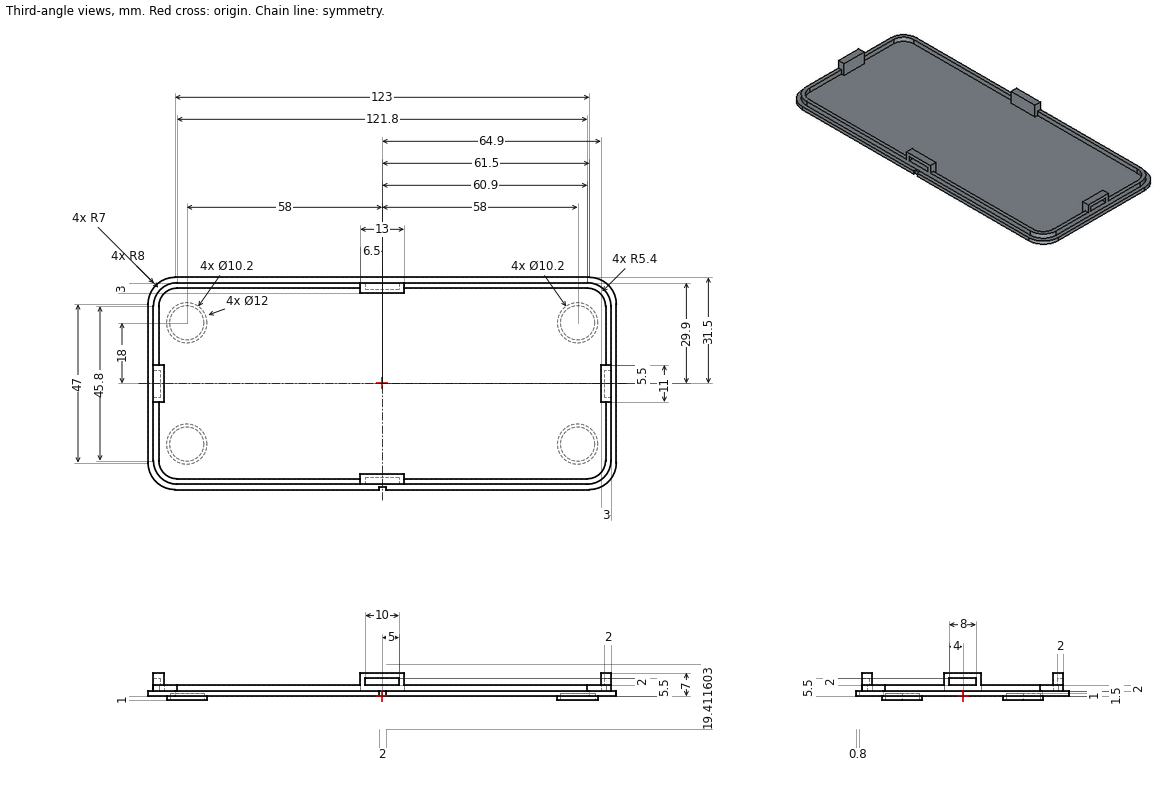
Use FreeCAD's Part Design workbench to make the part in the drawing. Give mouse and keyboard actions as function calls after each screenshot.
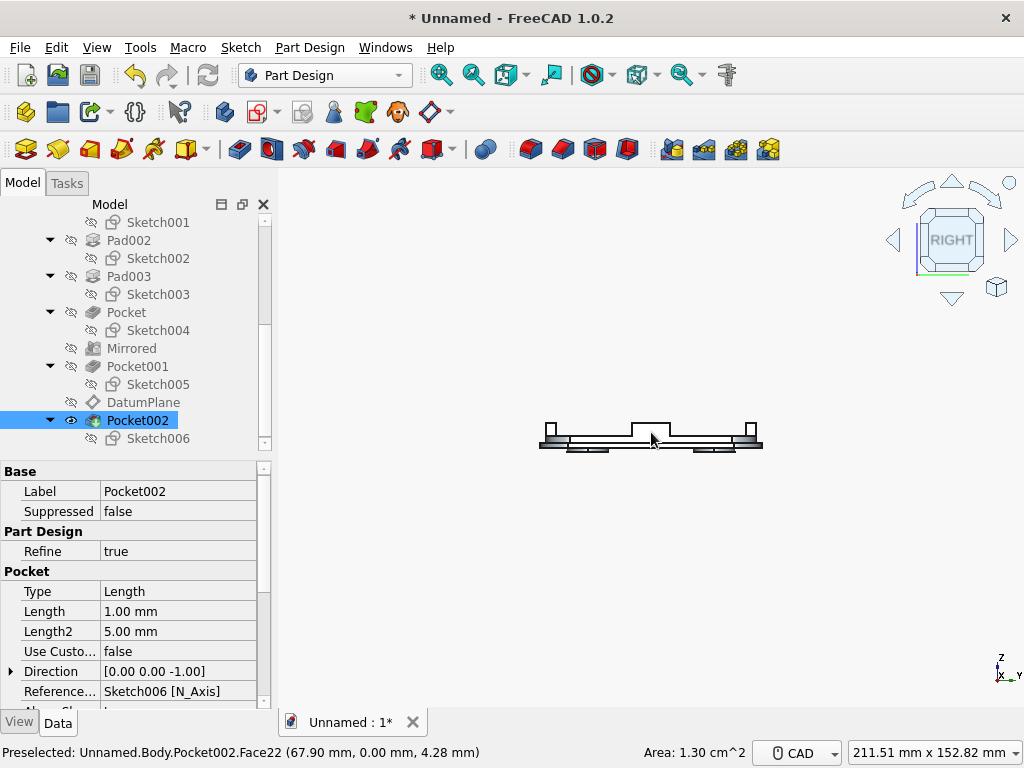
click(258, 112)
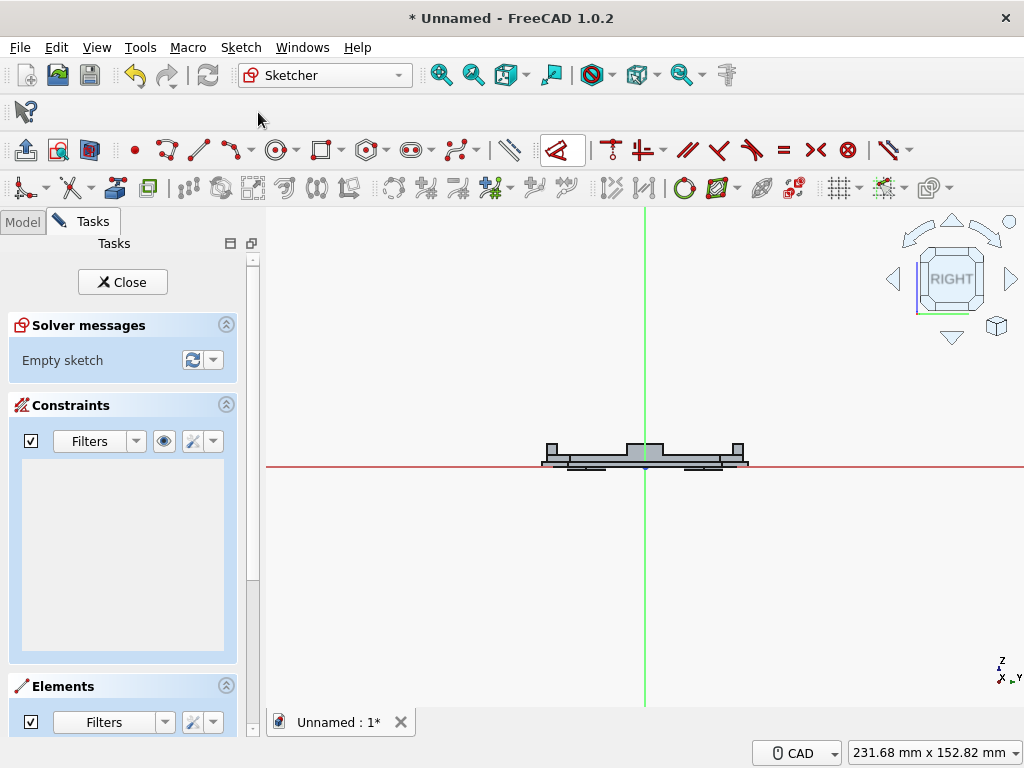
click(90, 150)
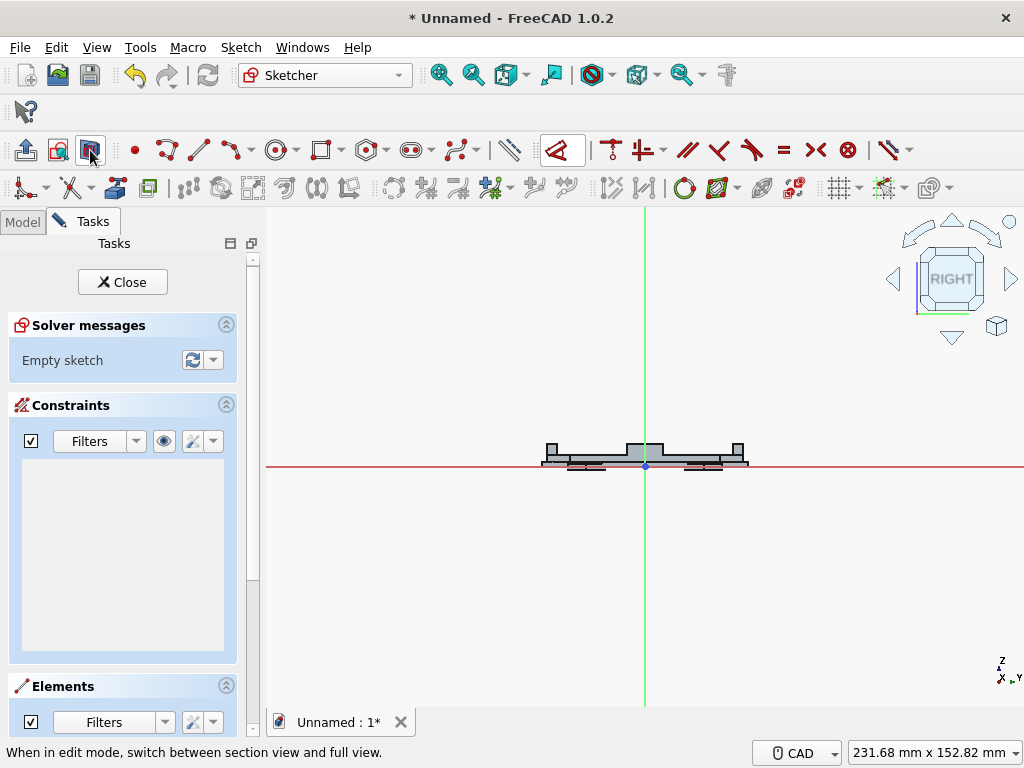
scroll(649, 458, up, 14)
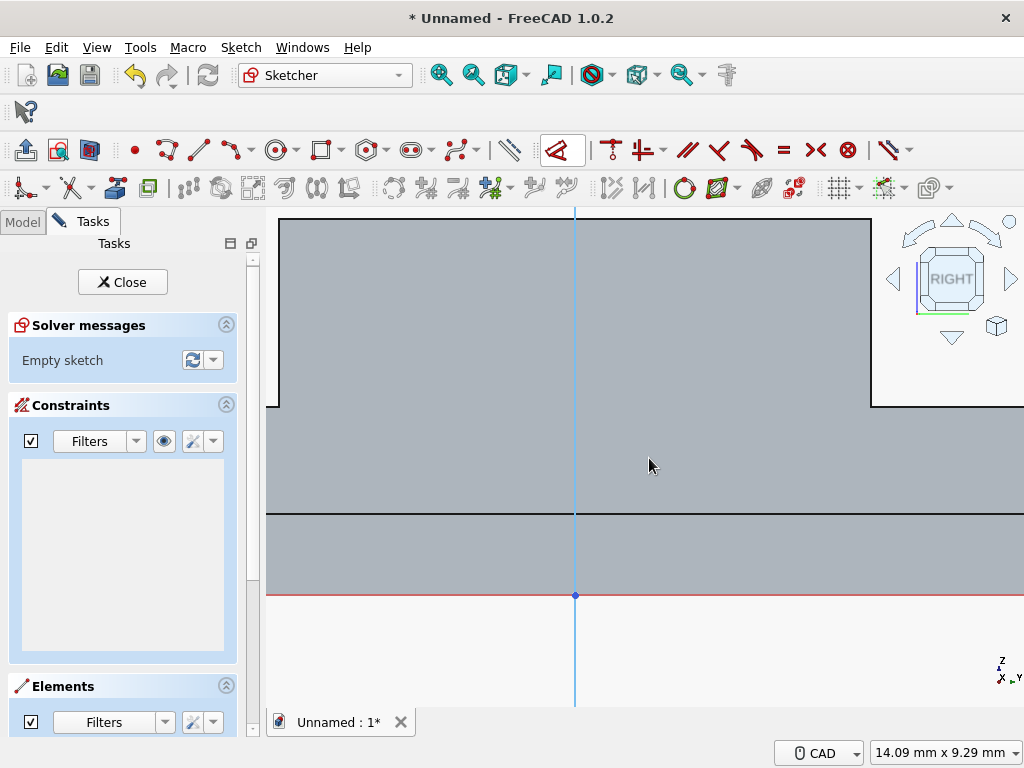
key(g)
key(r)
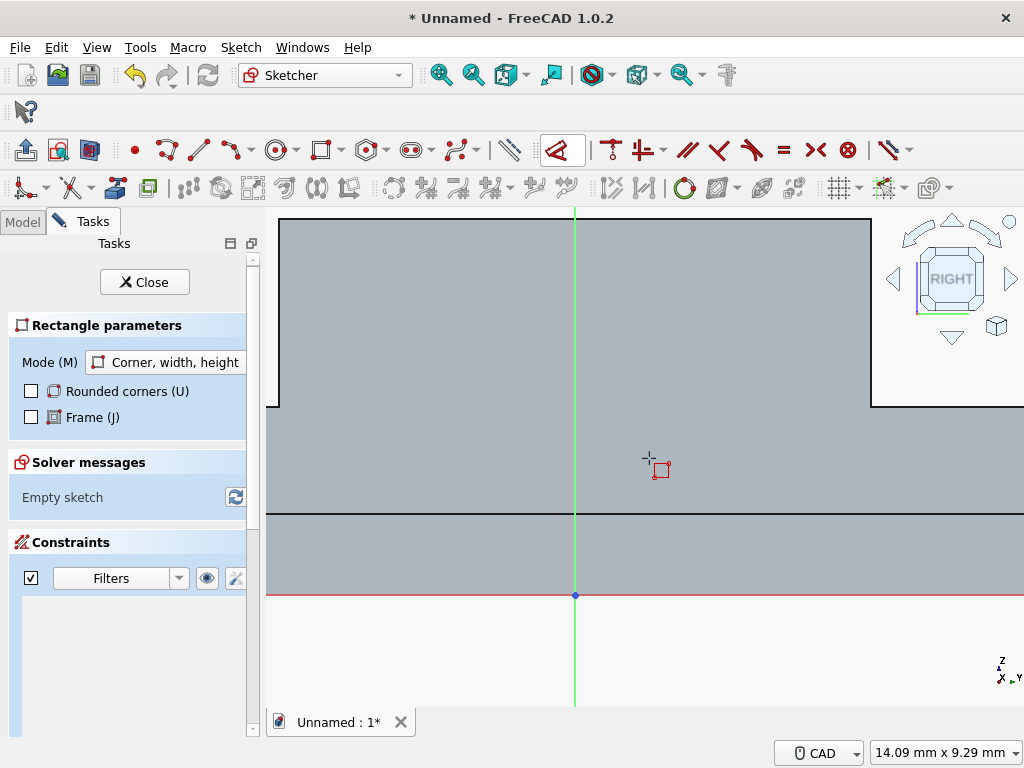
click(360, 299)
click(791, 407)
key(Escape)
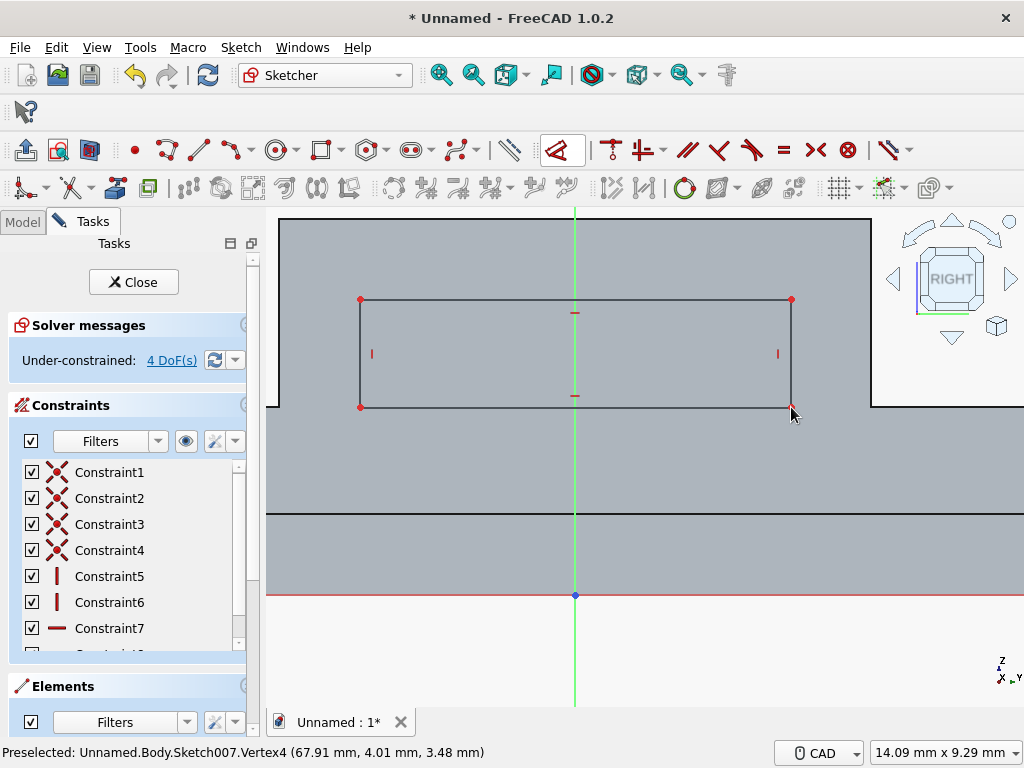
click(360, 332)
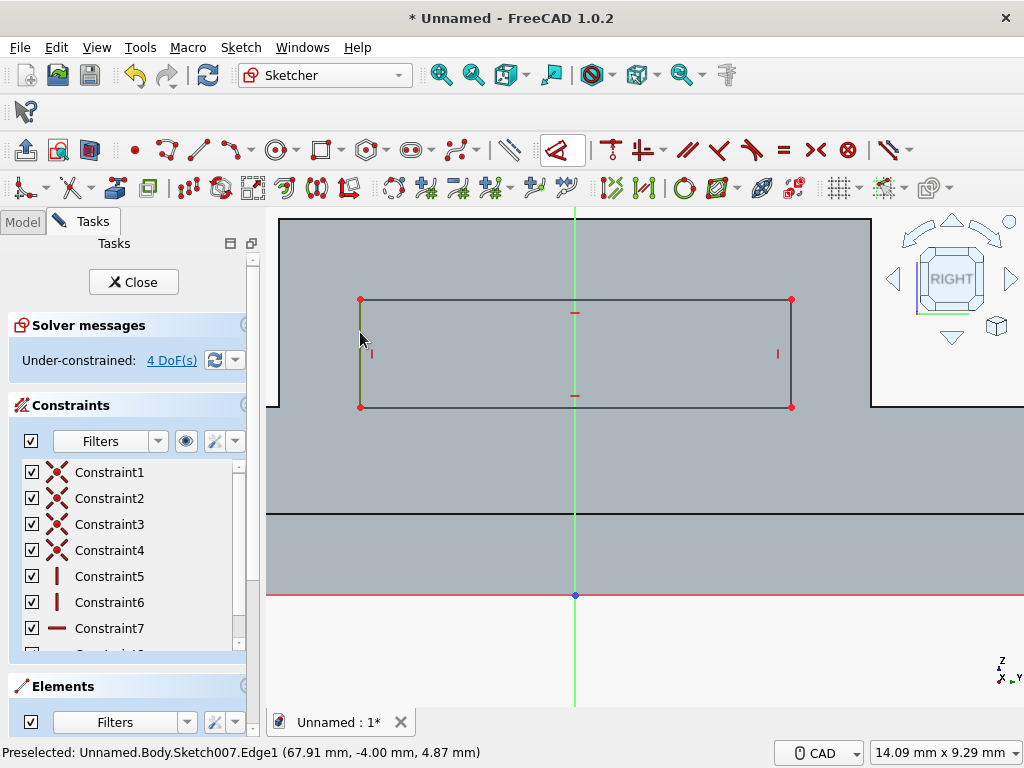
key(i)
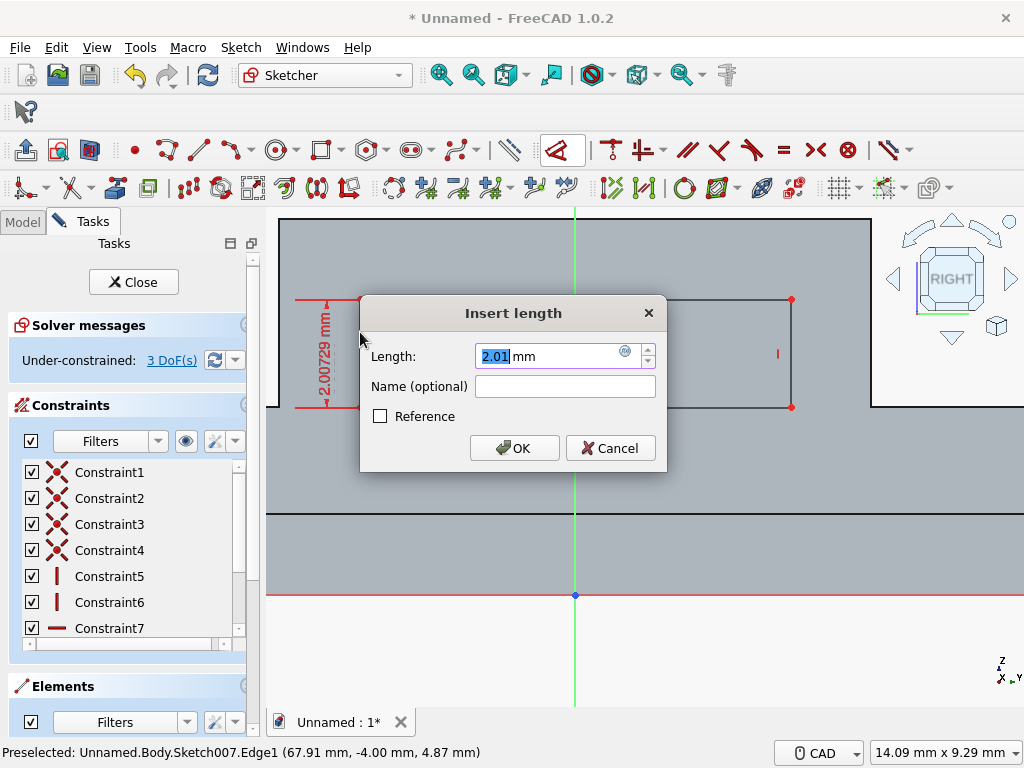
text(2)
key(Return)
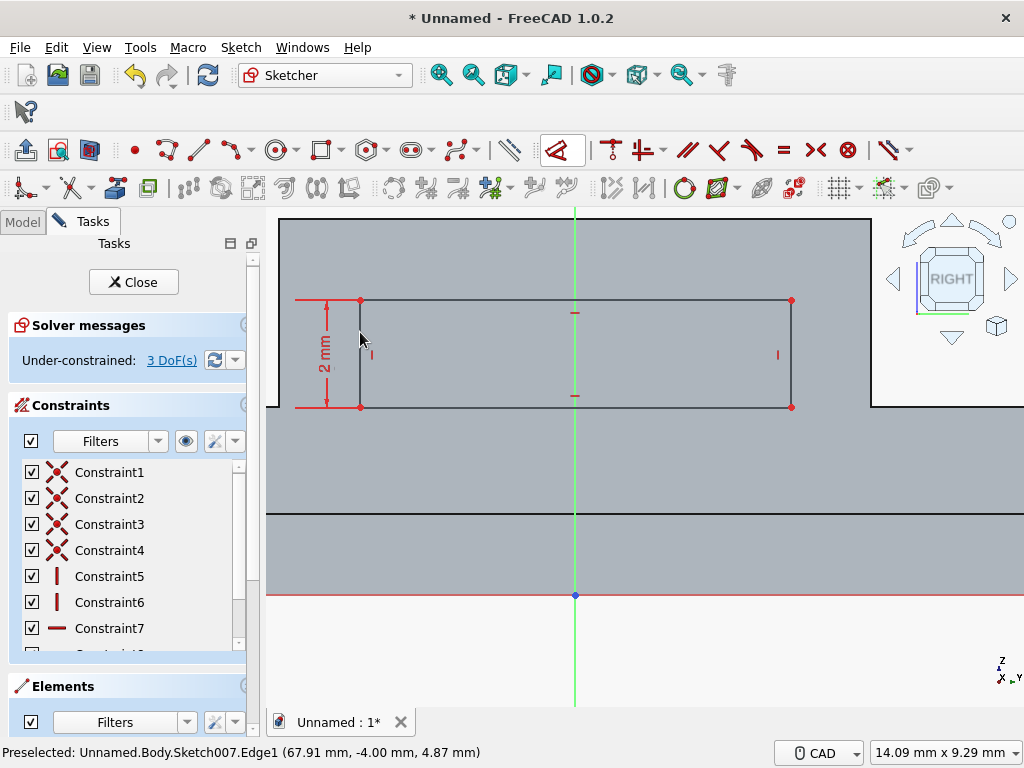
click(489, 408)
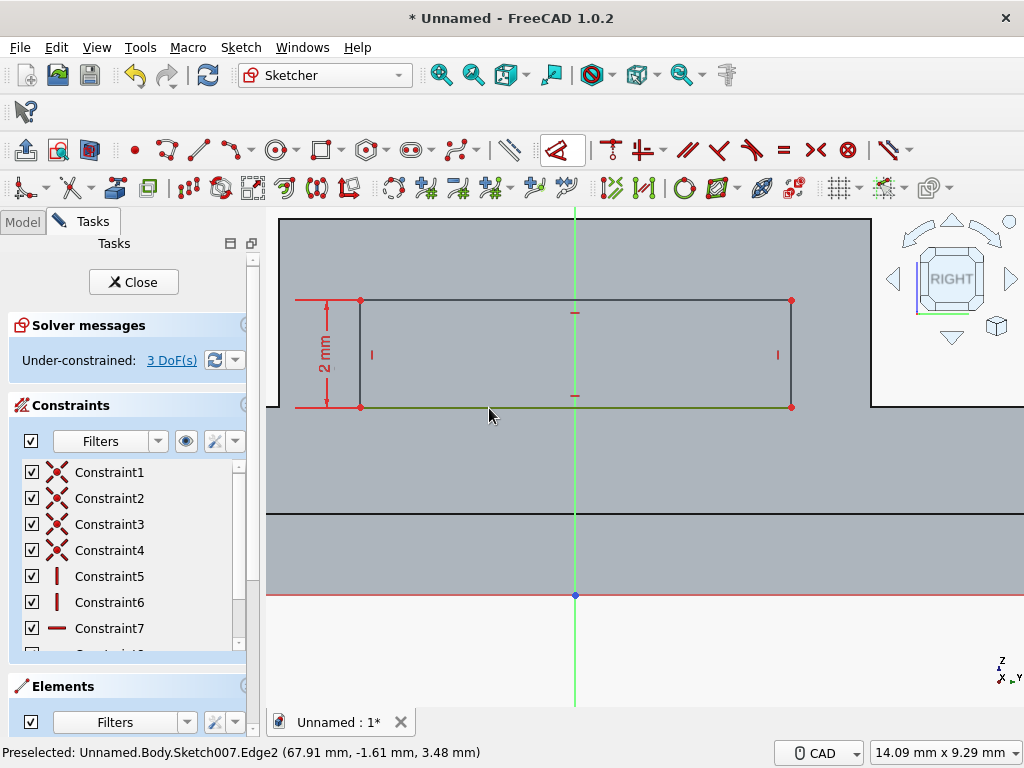
key(l)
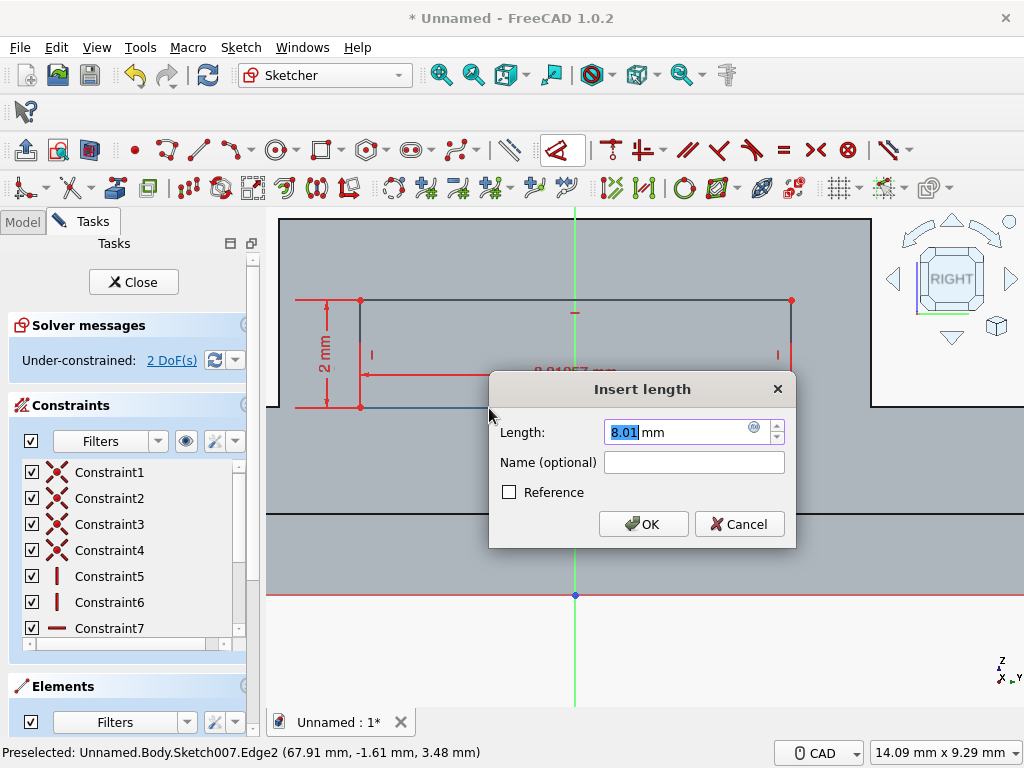
text(8)
key(Return)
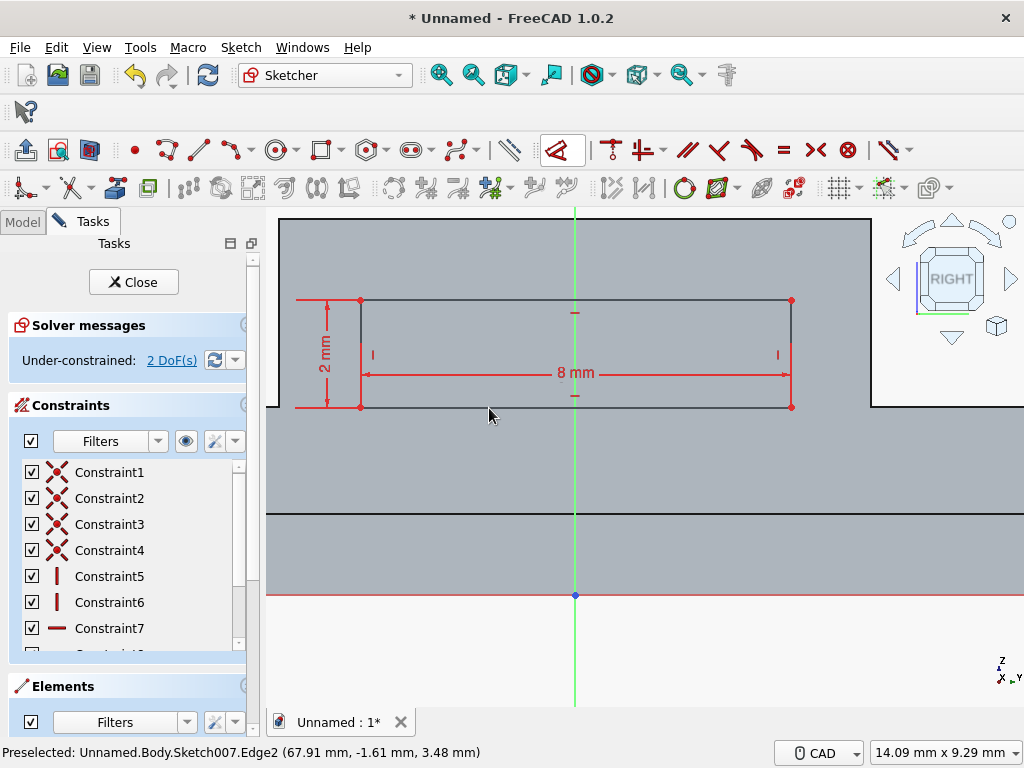
click(361, 300)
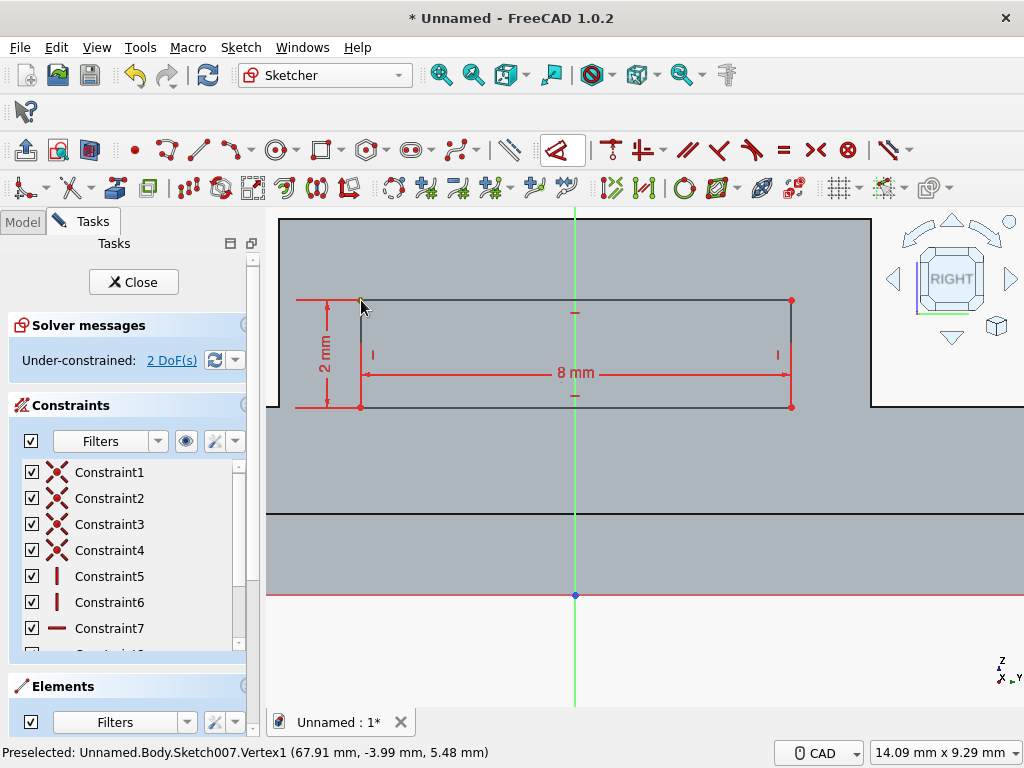
key(l)